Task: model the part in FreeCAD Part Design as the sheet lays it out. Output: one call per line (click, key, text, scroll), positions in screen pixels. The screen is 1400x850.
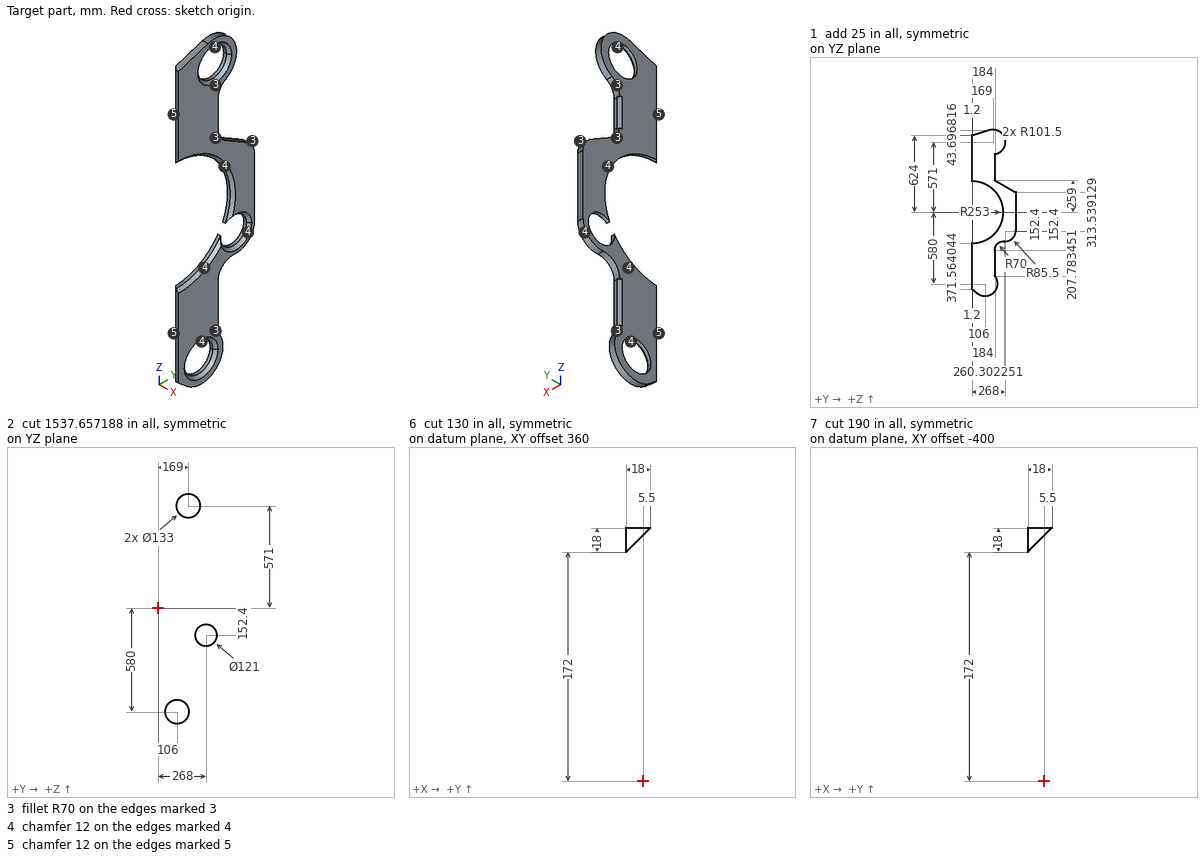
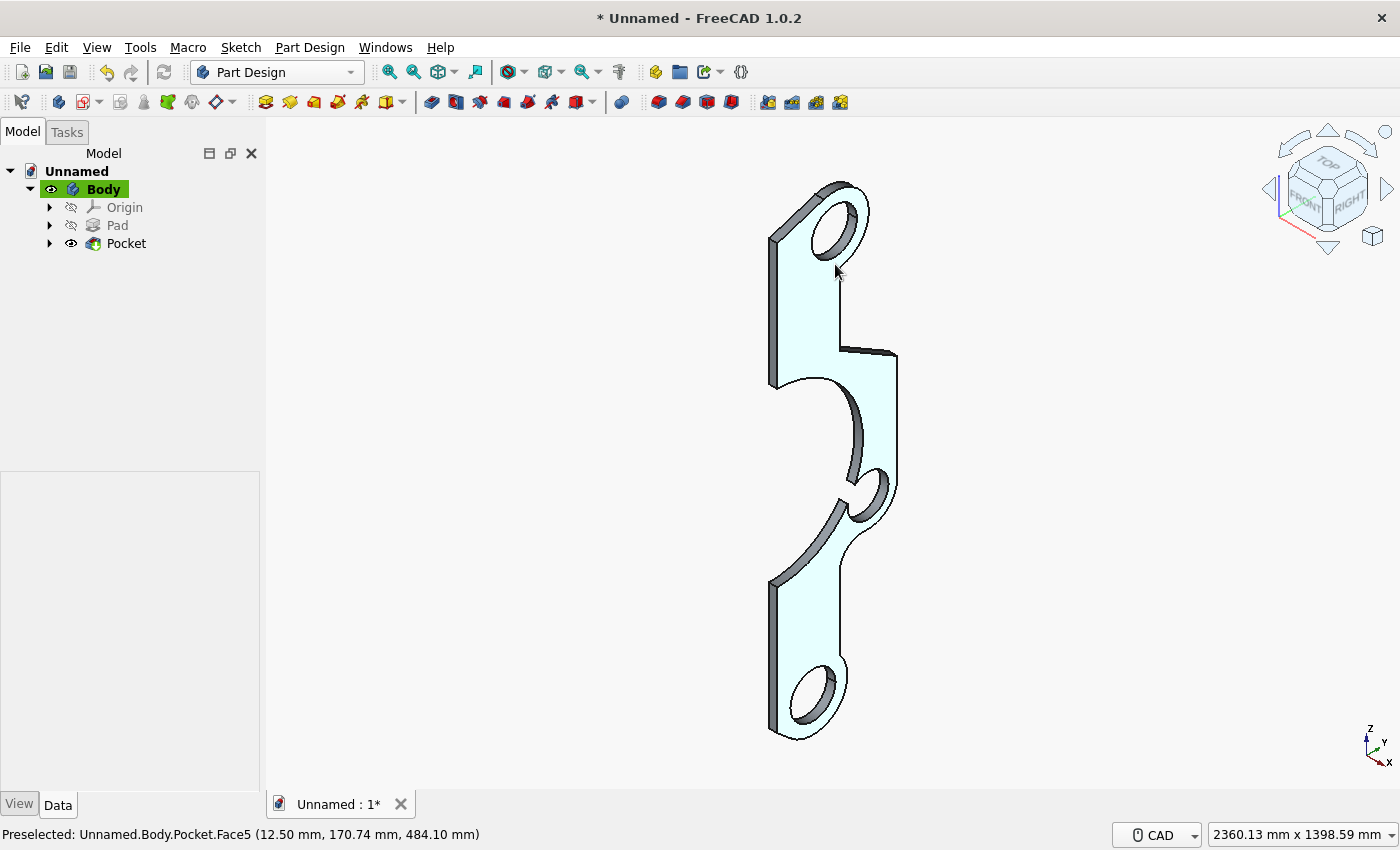
key(2)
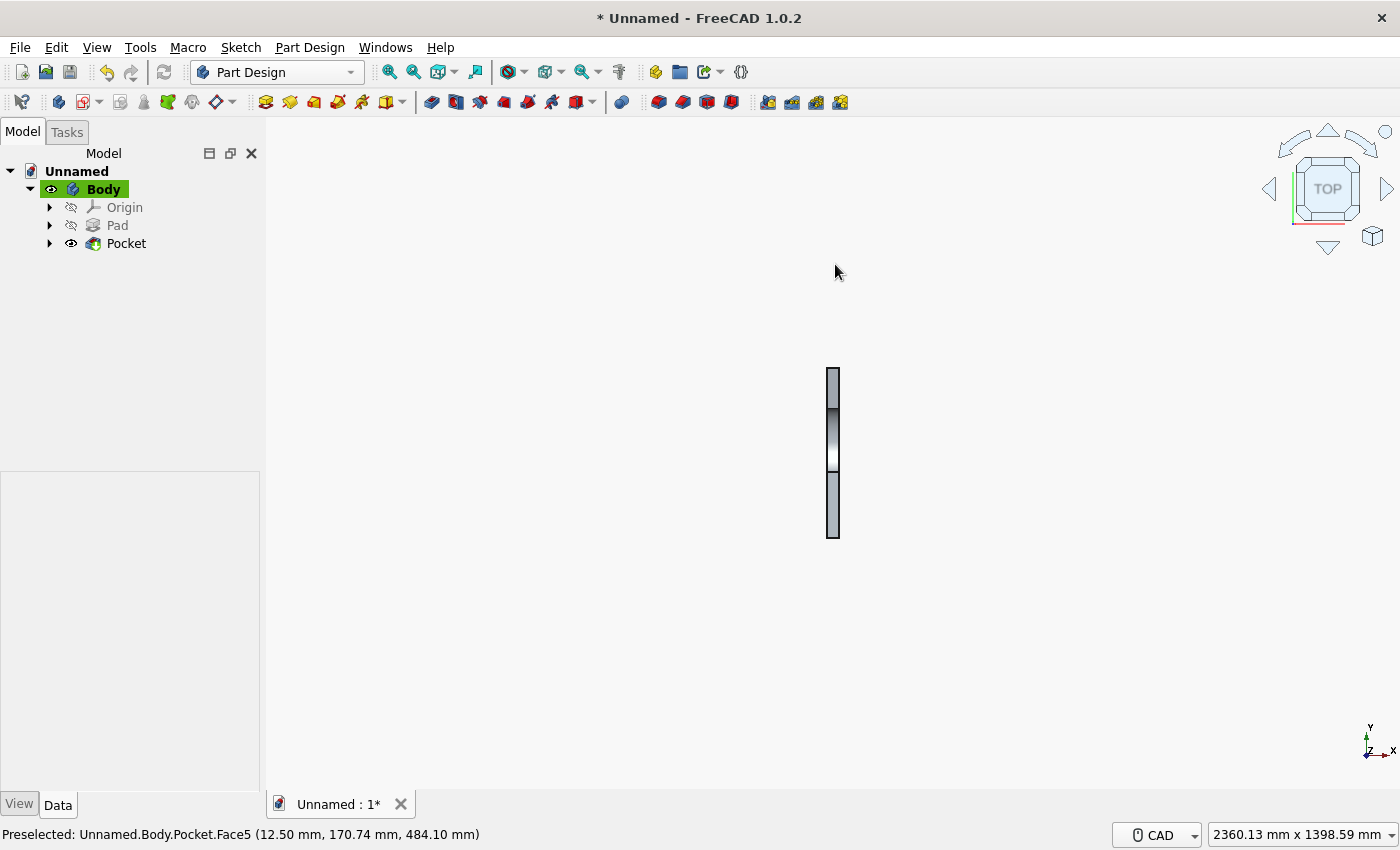
click(390, 72)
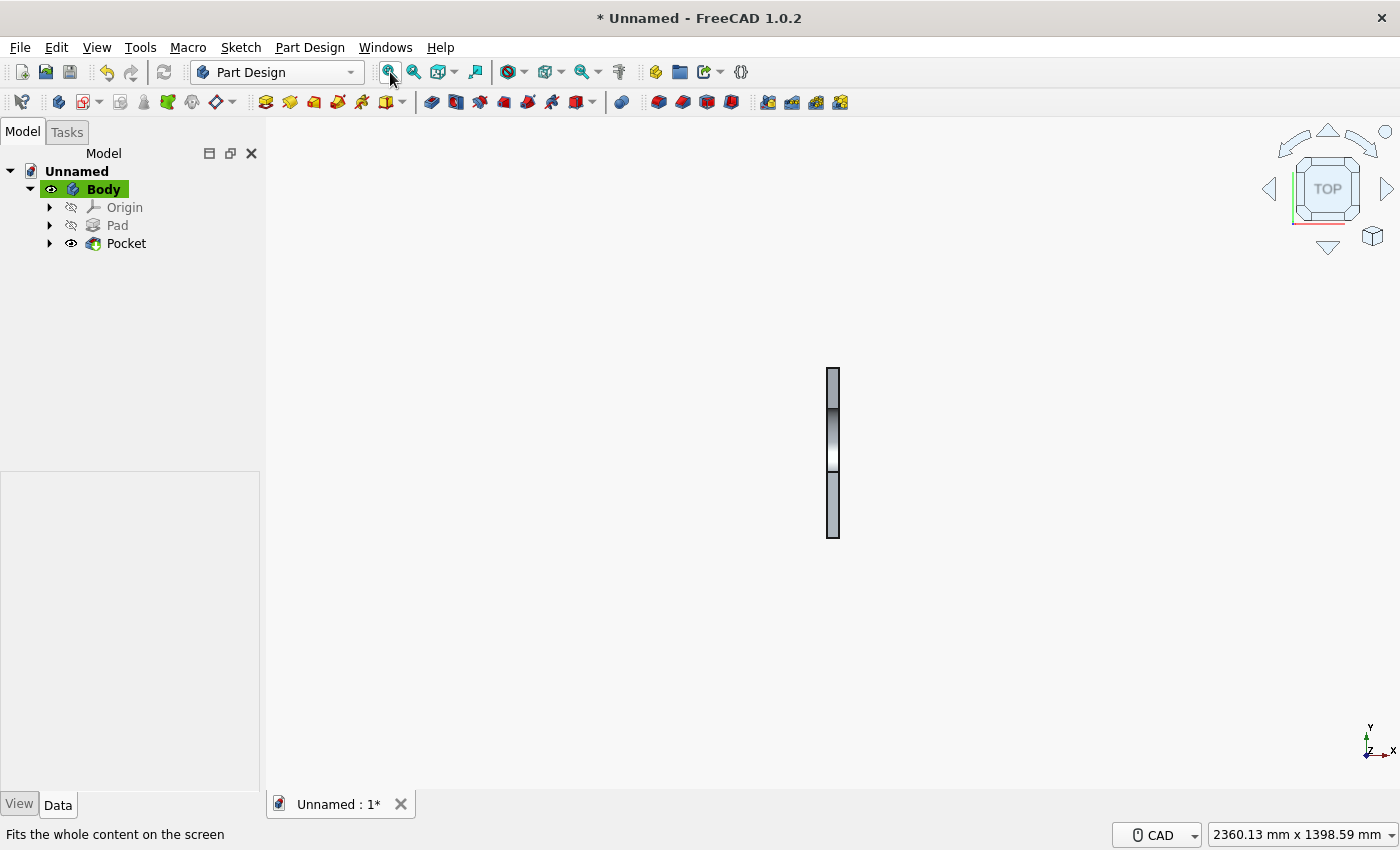
scroll(833, 449, up, 7)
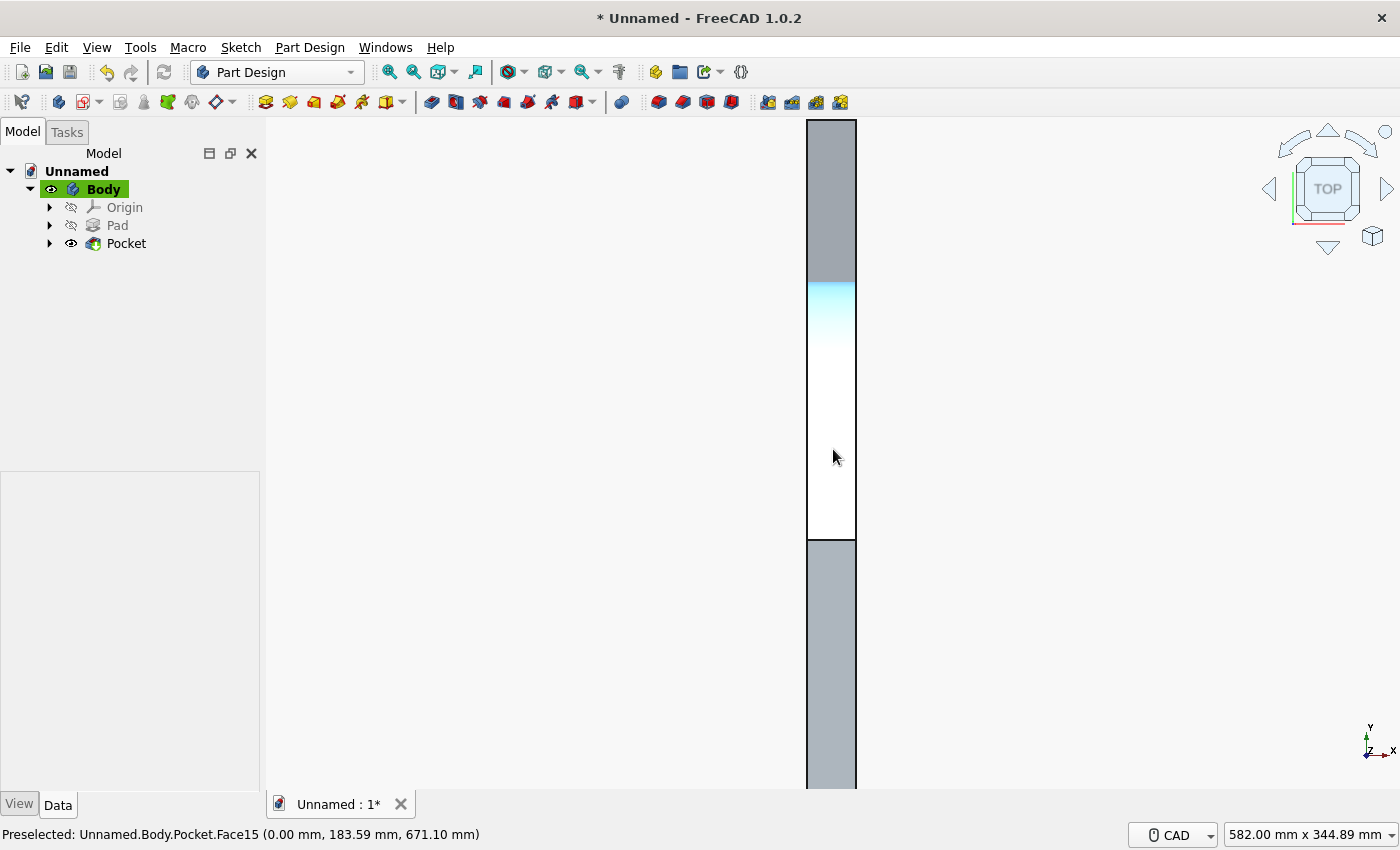
key(v)
key(f)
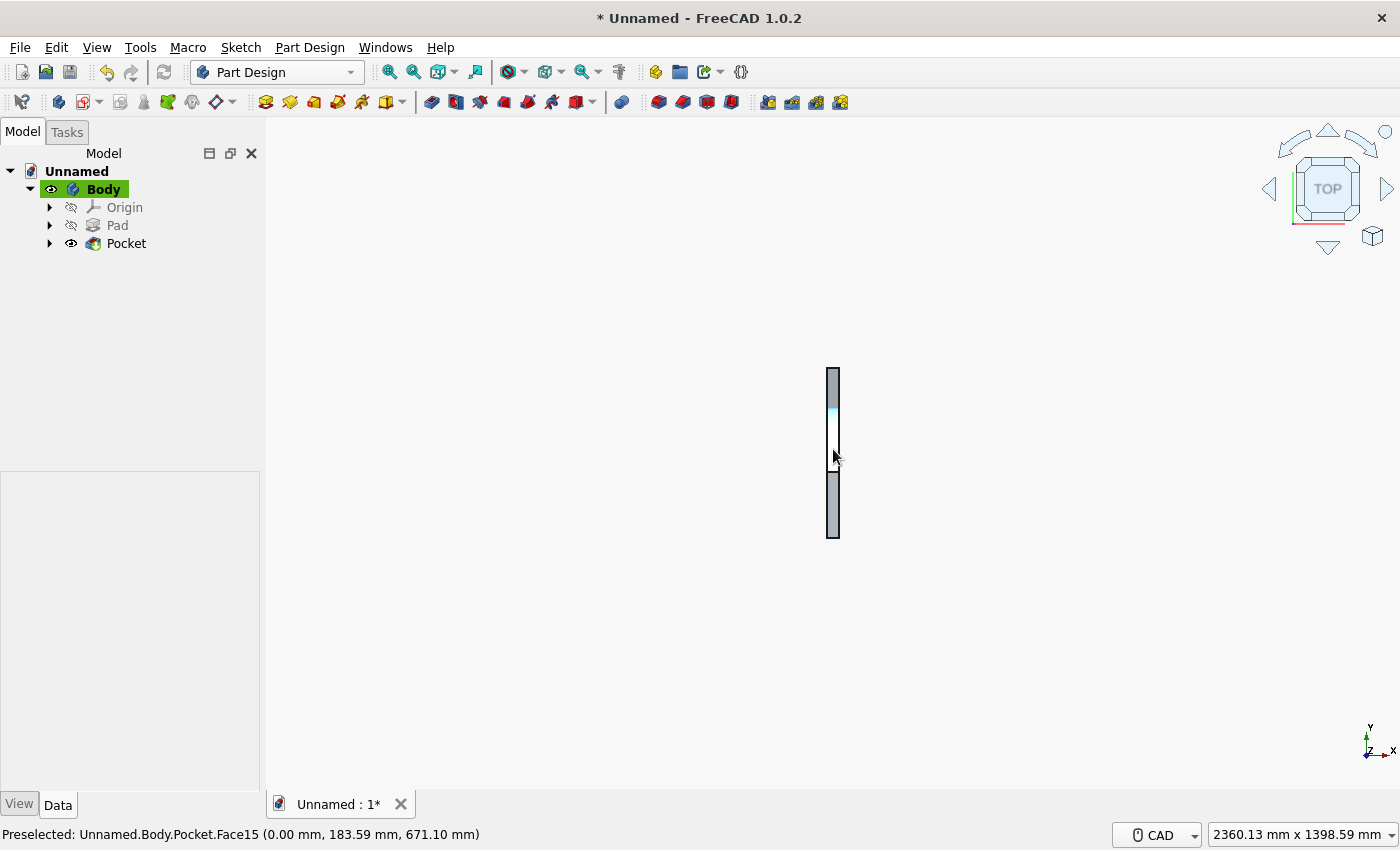
key(1)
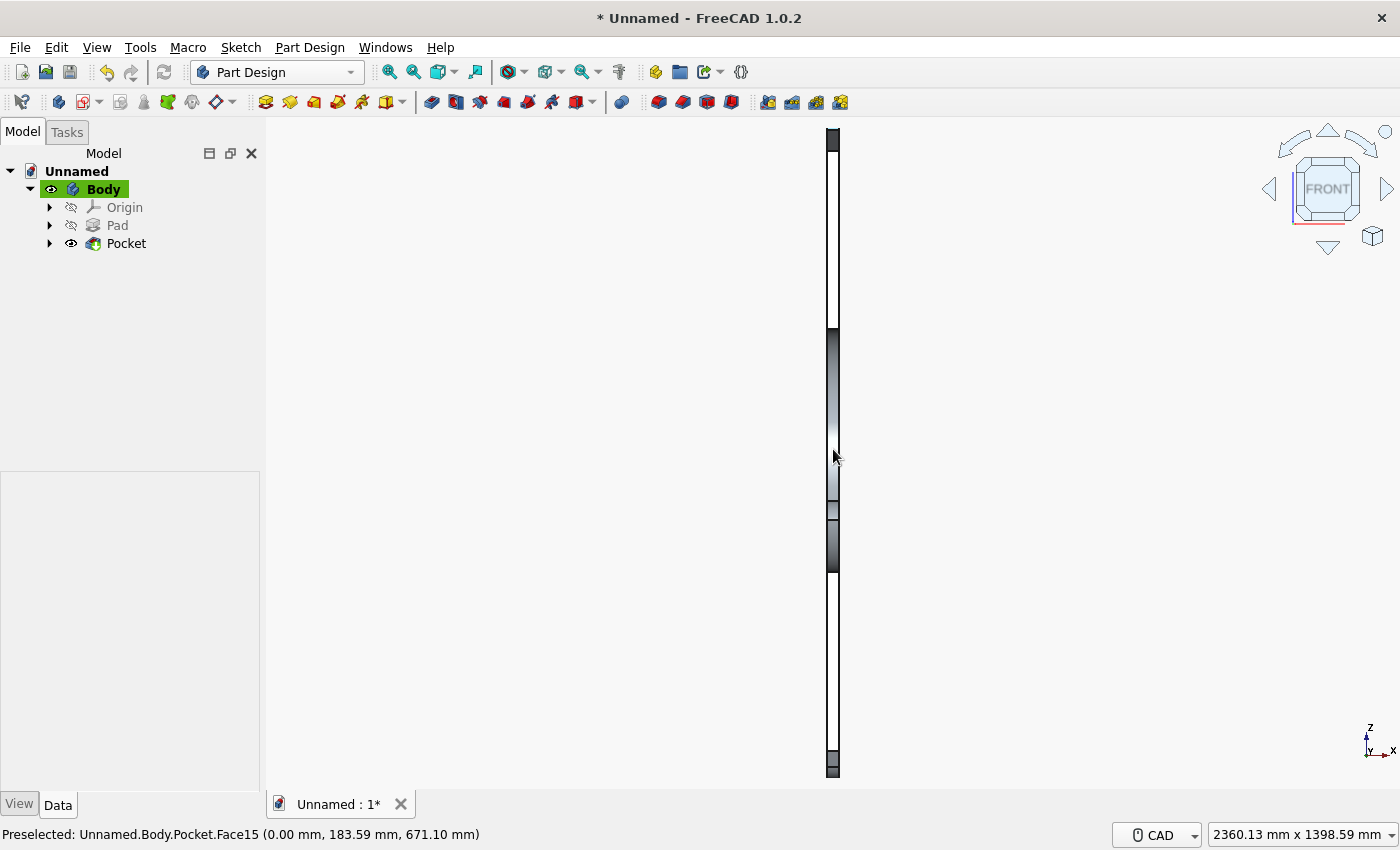
scroll(833, 224, up, 7)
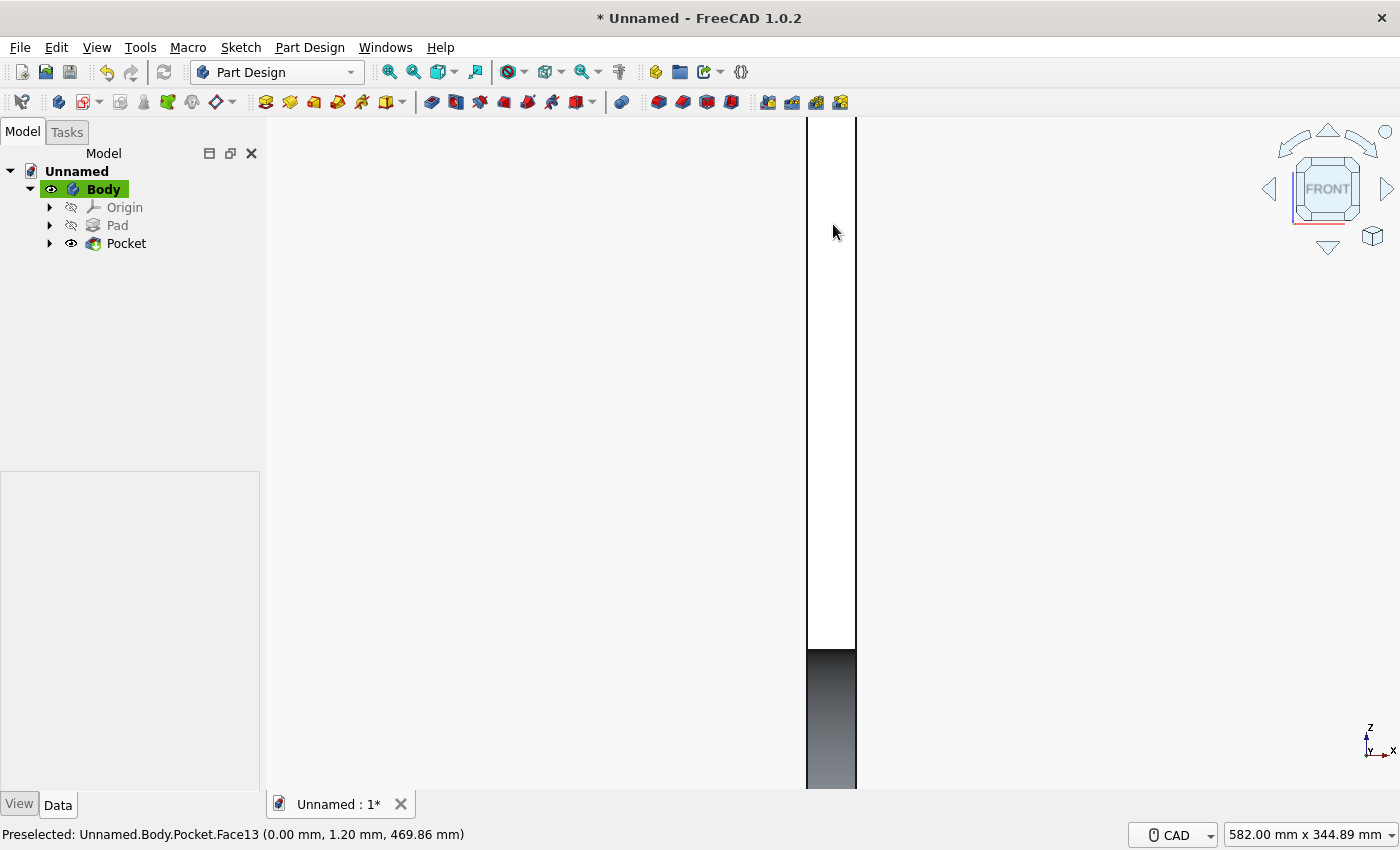
key(v)
key(f)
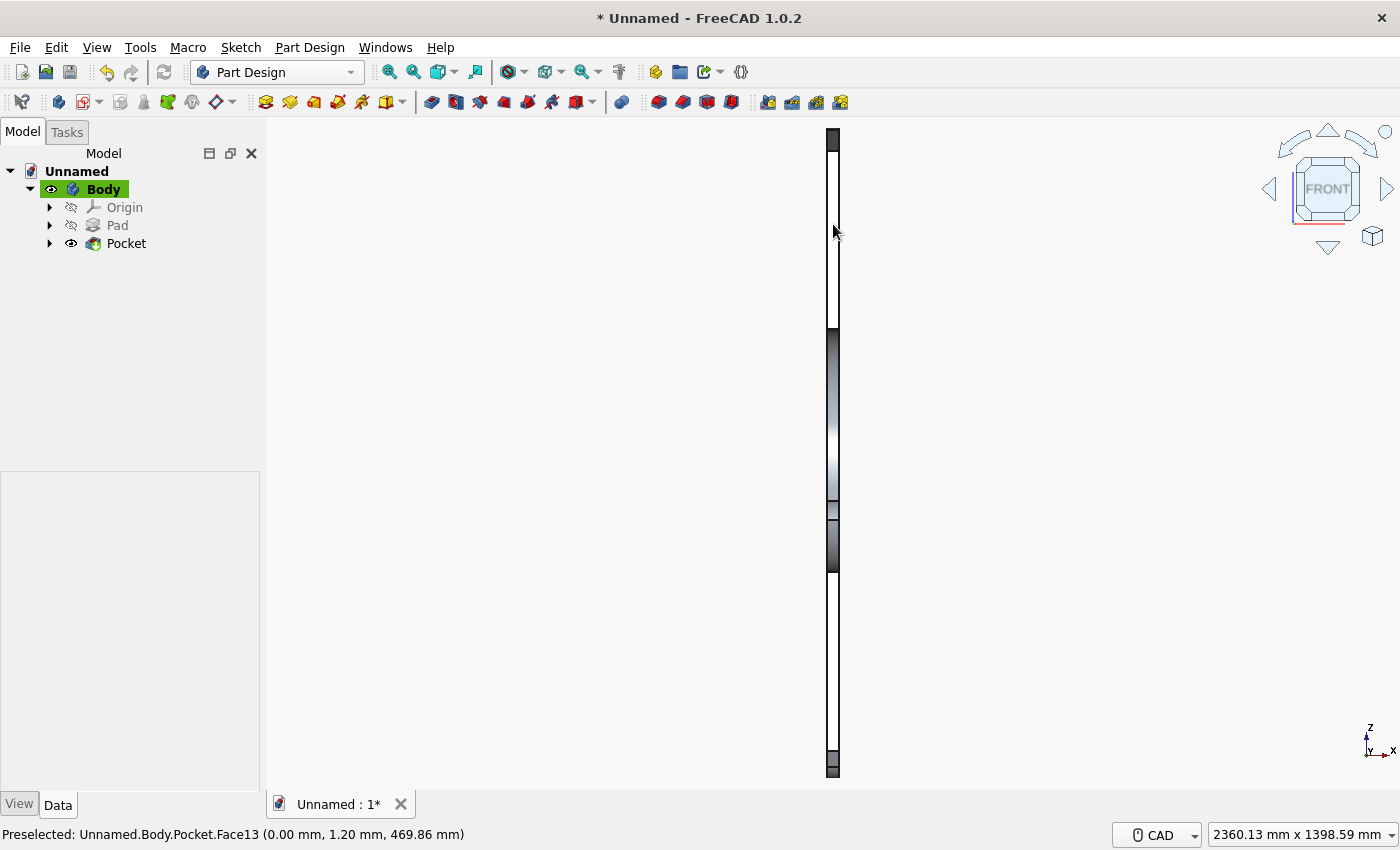
key(3)